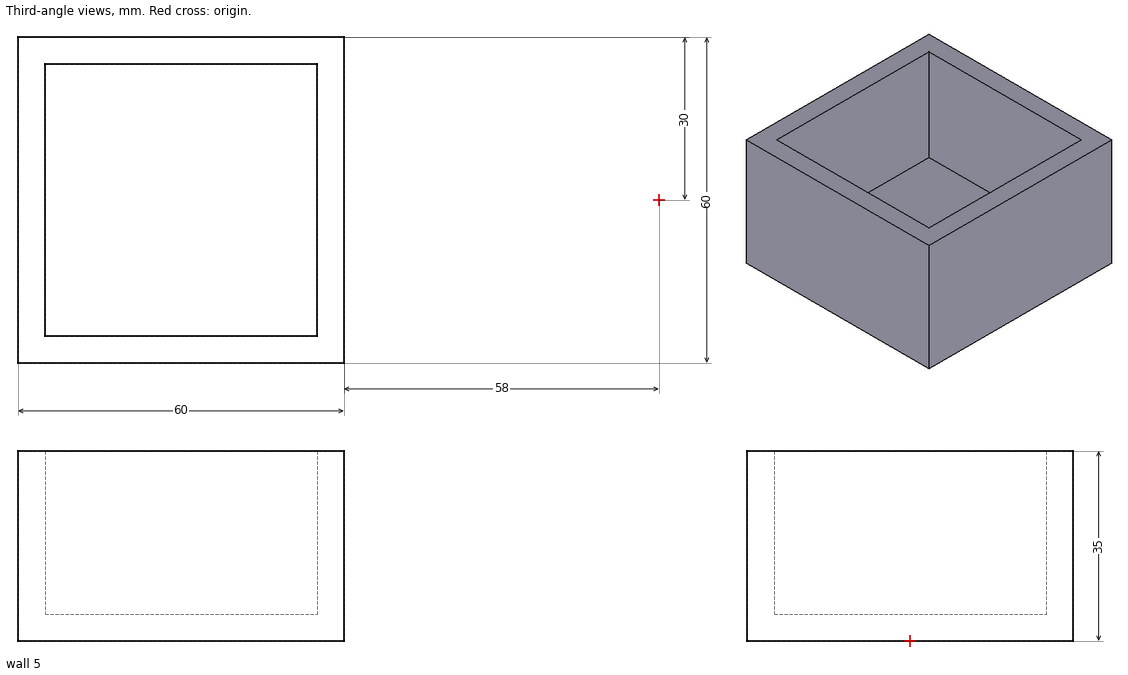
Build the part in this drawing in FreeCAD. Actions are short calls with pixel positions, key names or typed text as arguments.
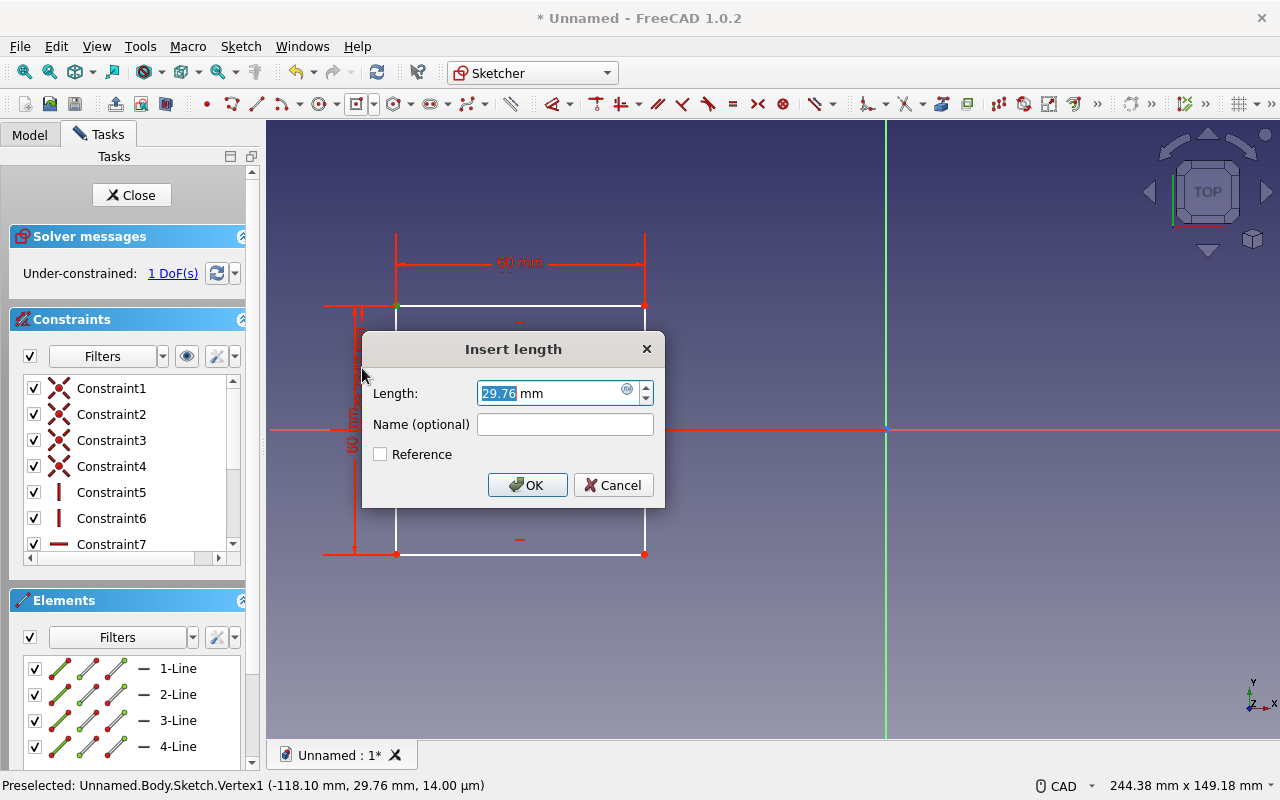
text(30)
key(Return)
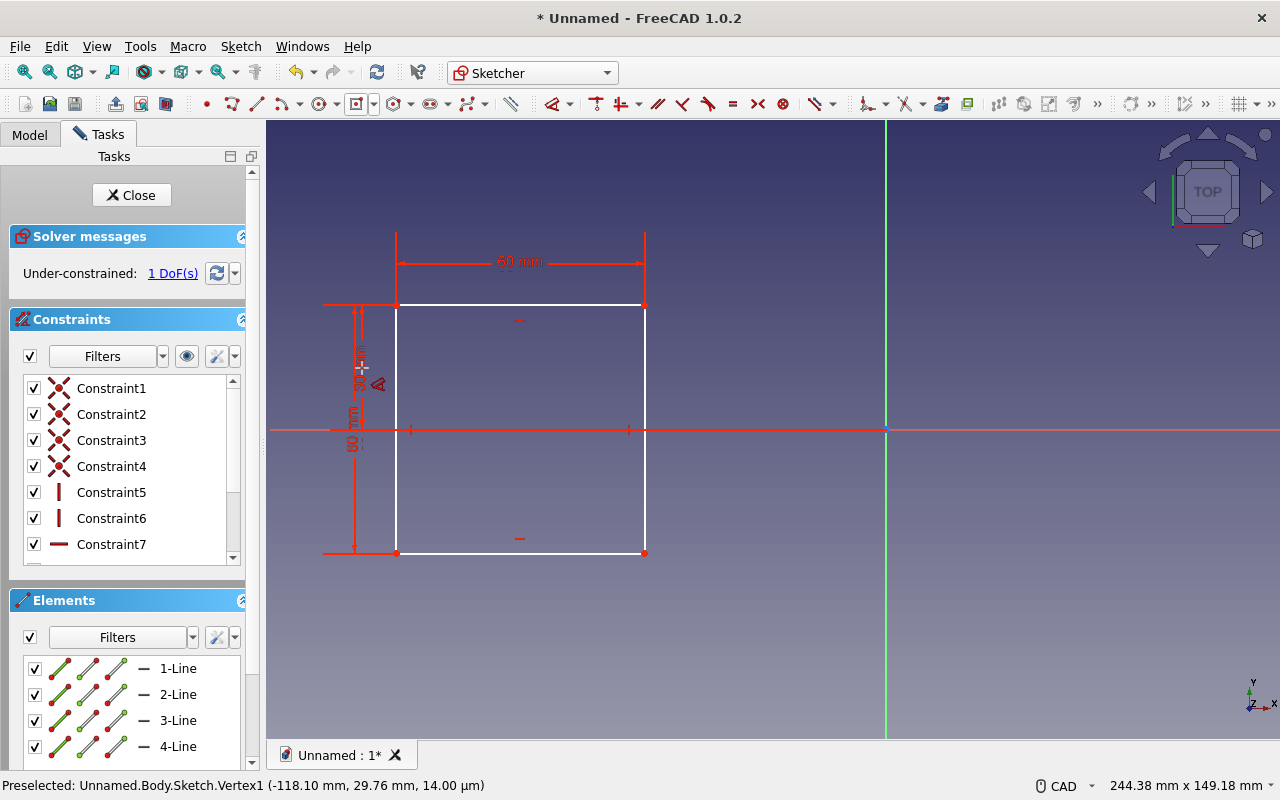
click(645, 554)
click(765, 588)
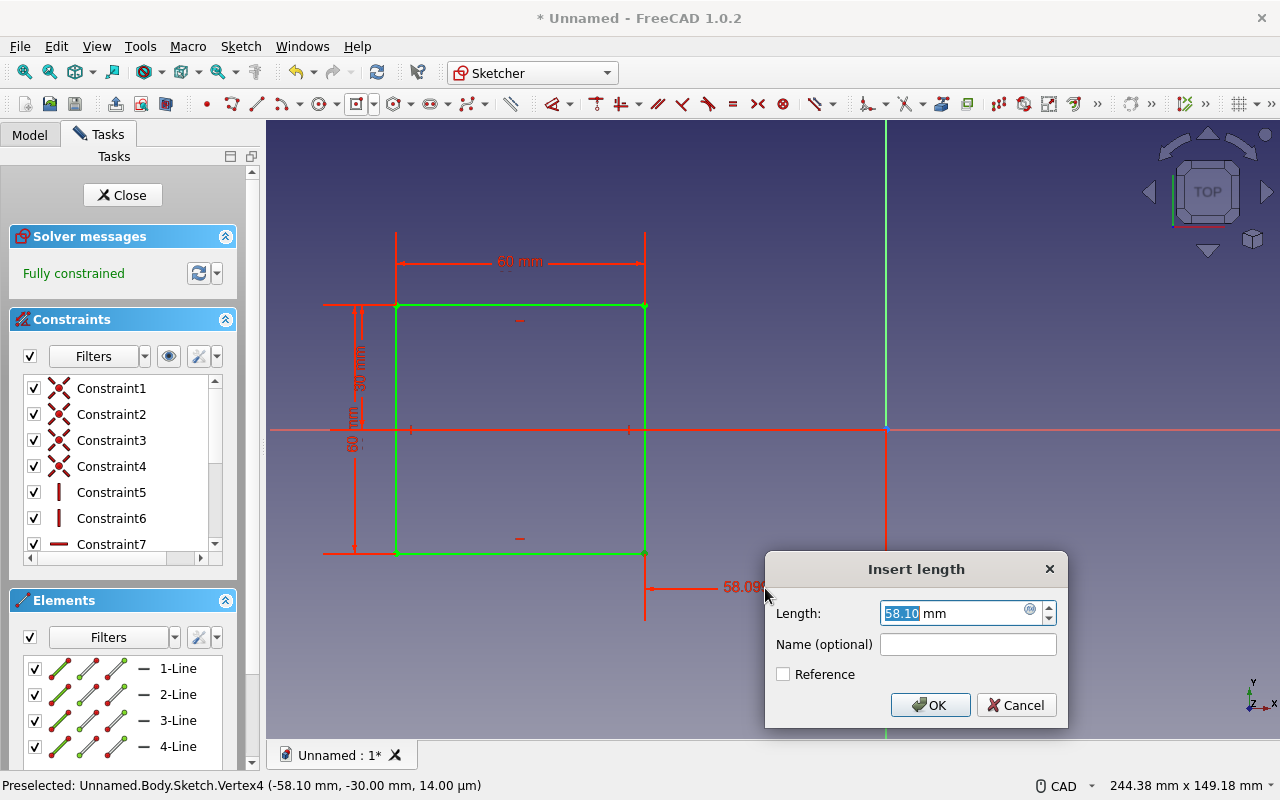
text(58)
key(Return)
key(Escape)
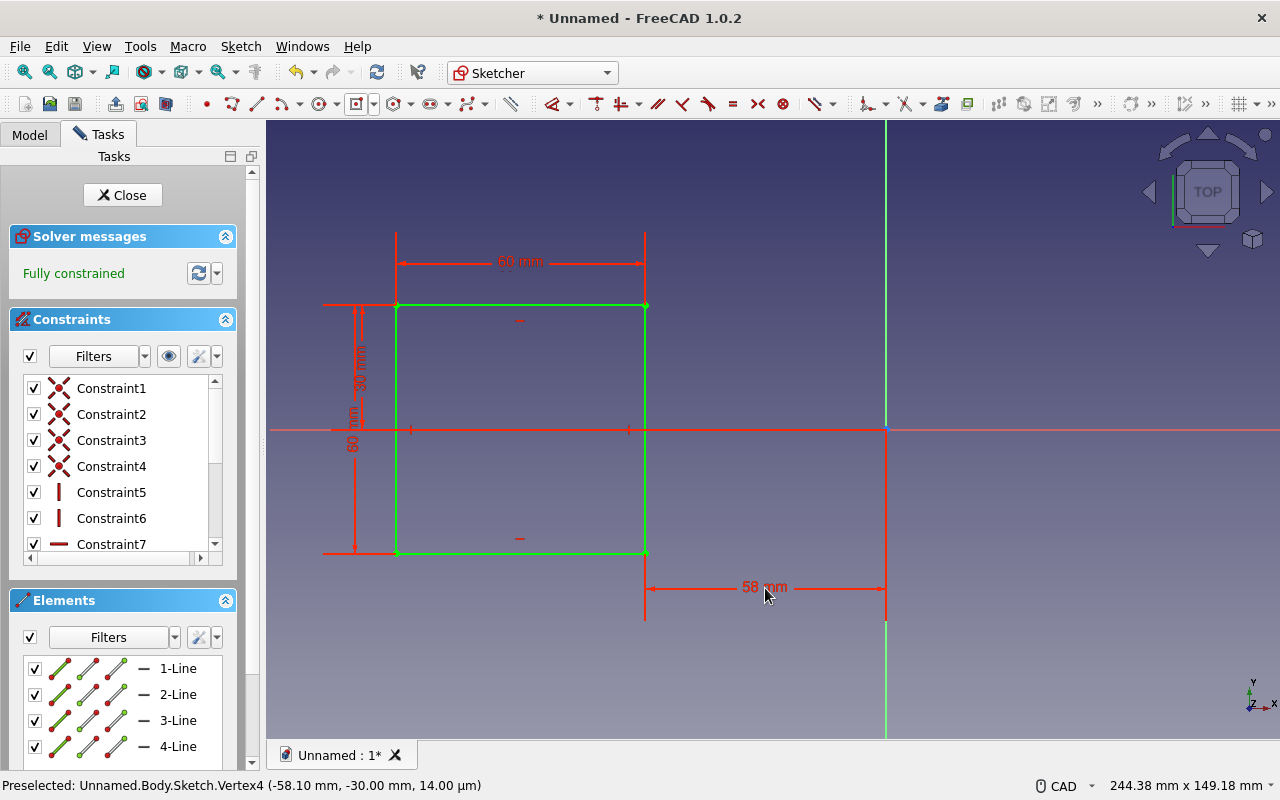
click(123, 195)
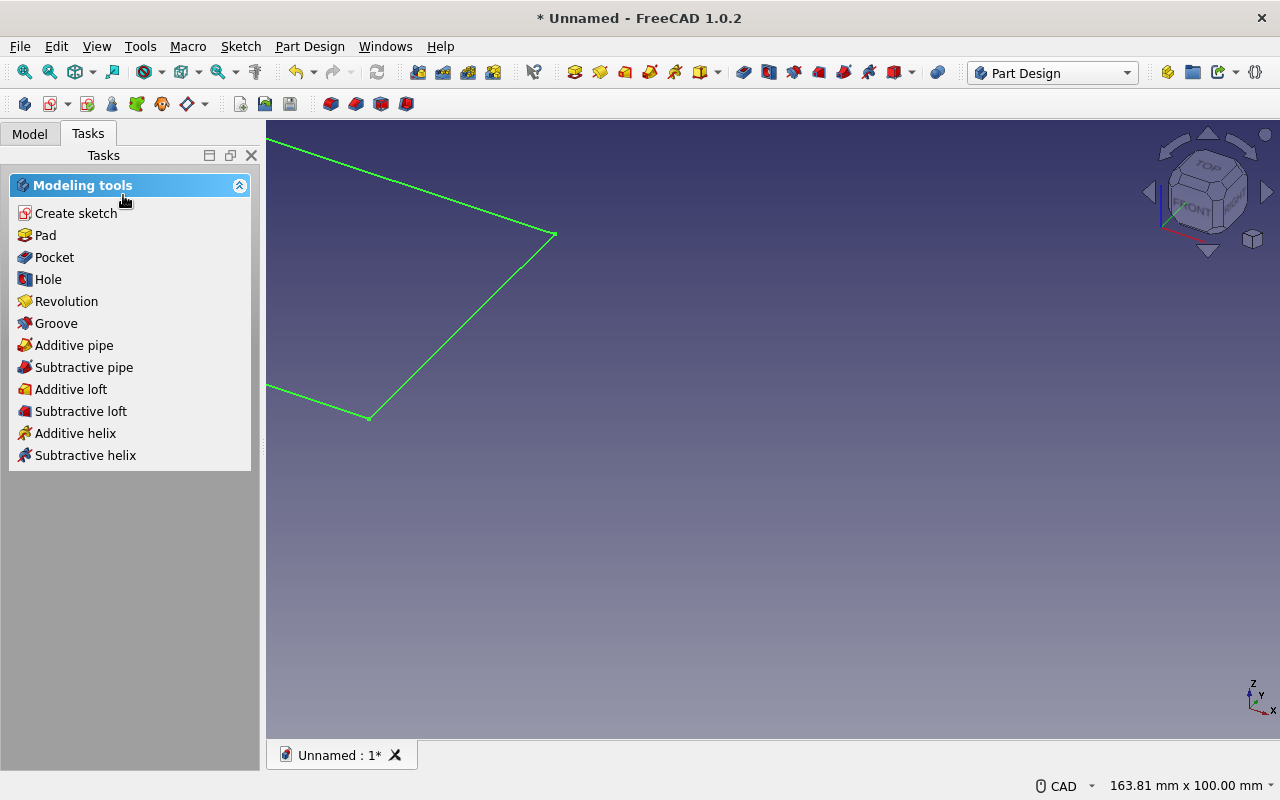
click(575, 72)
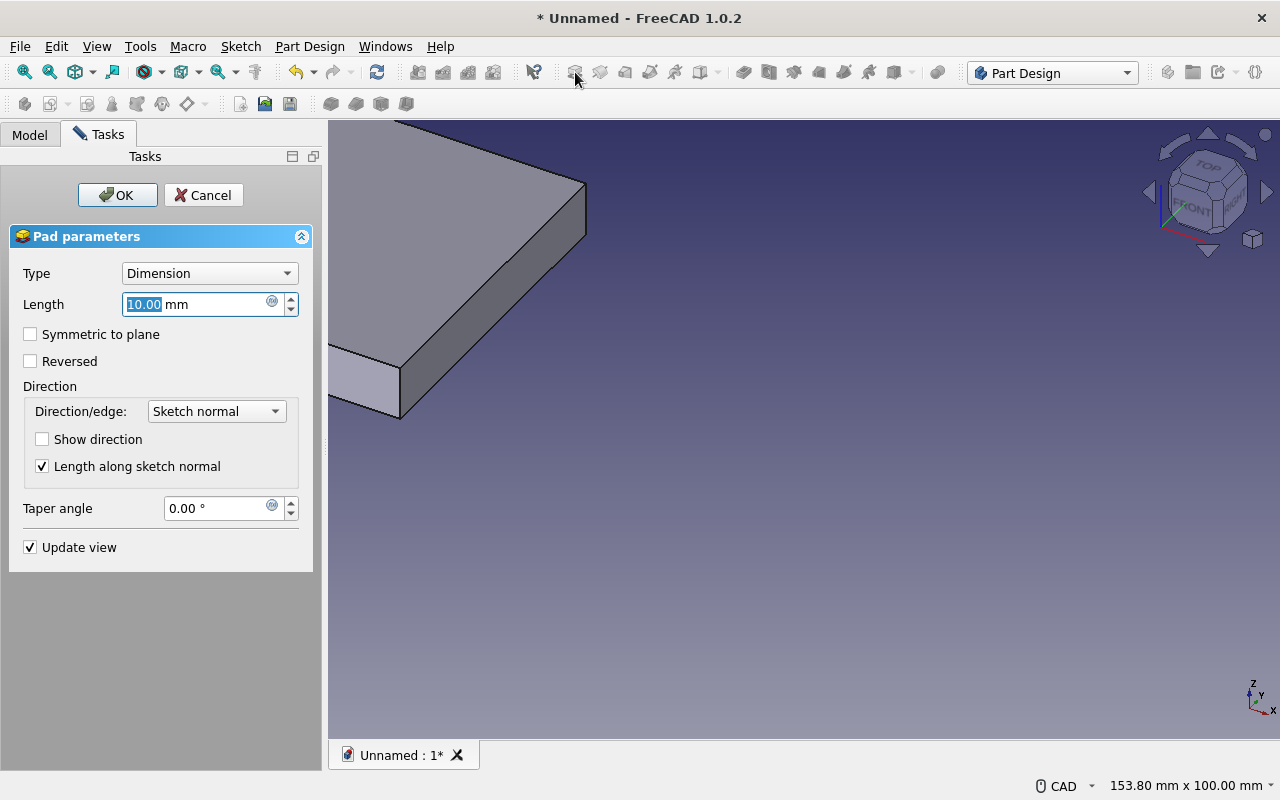
text(35)
key(Tab)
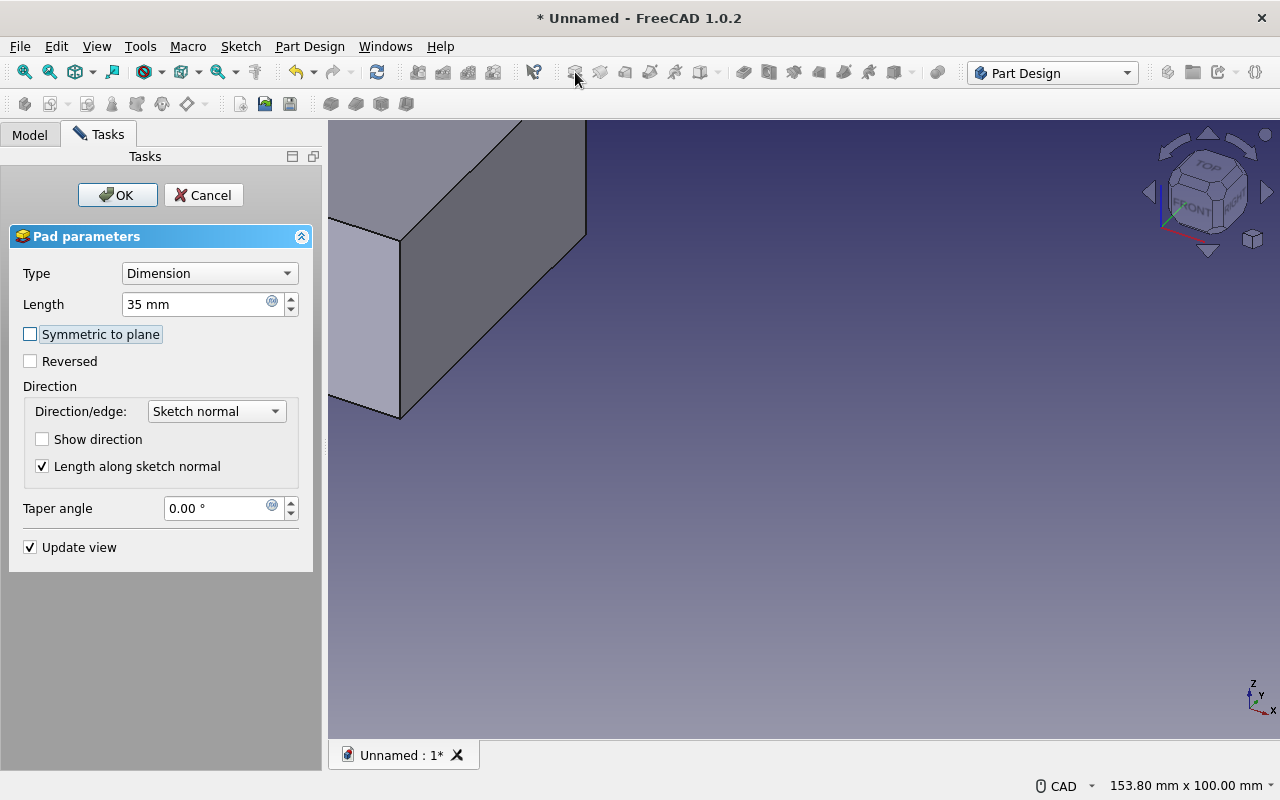
click(118, 195)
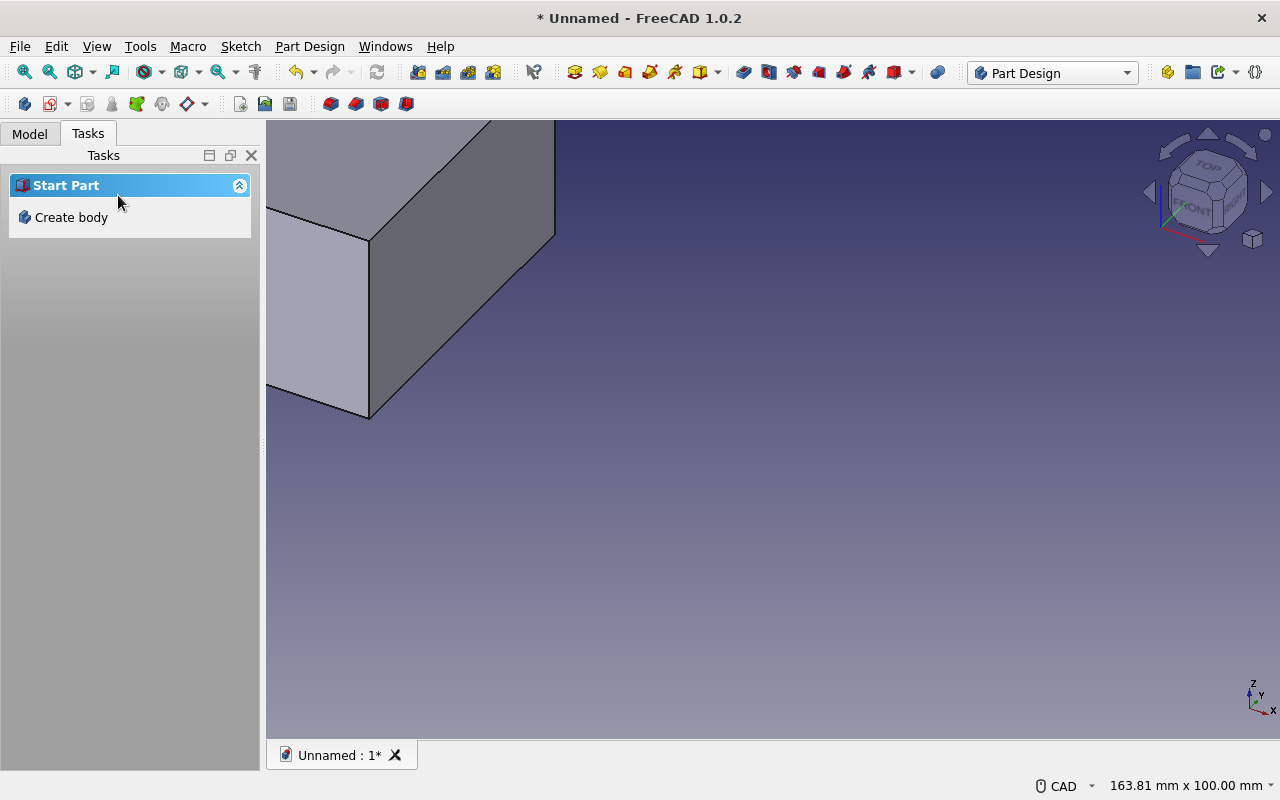
click(25, 72)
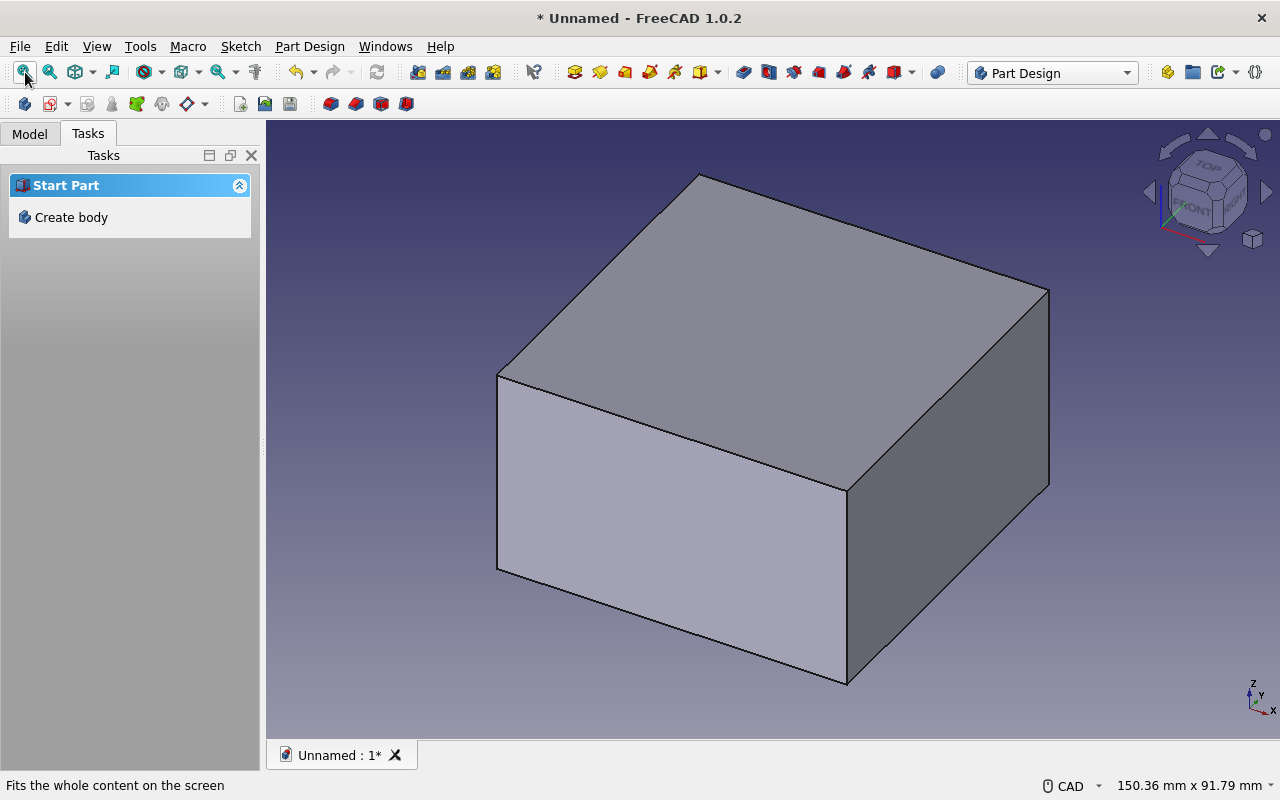
click(773, 332)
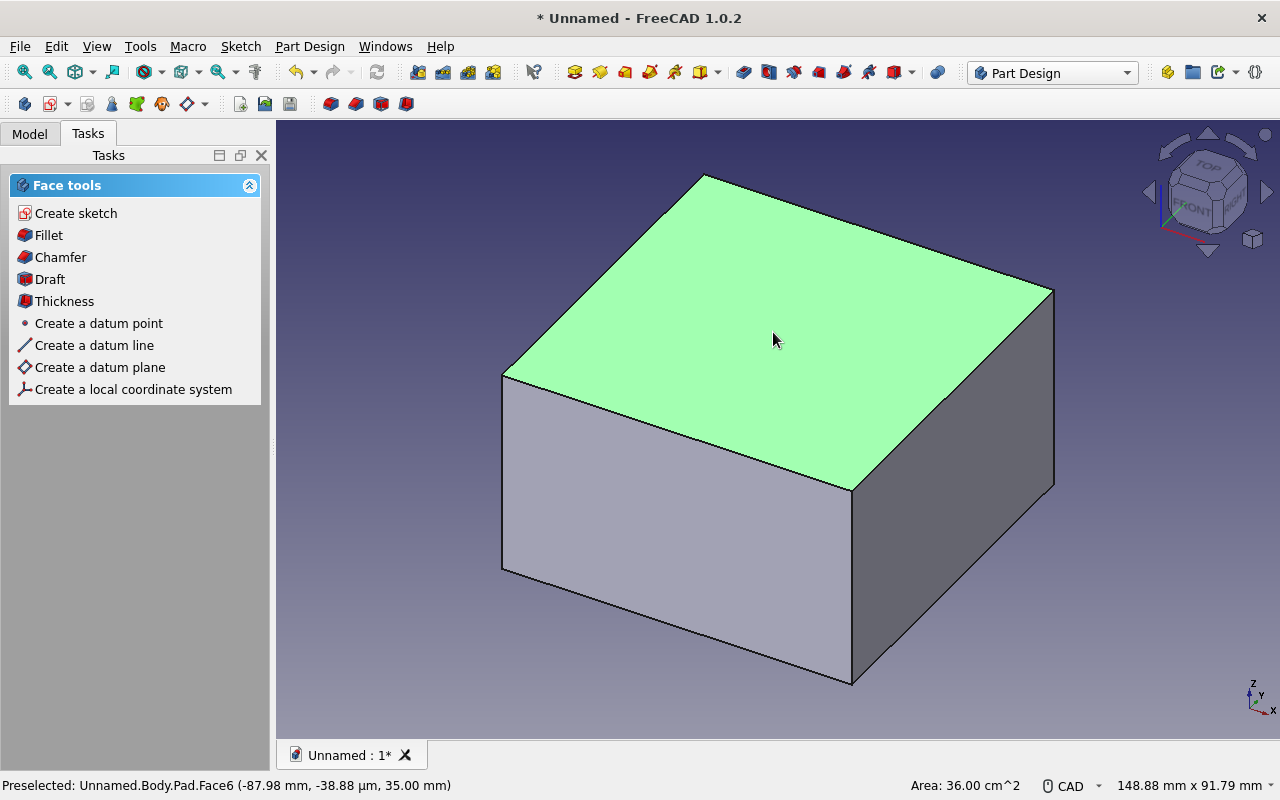
click(406, 104)